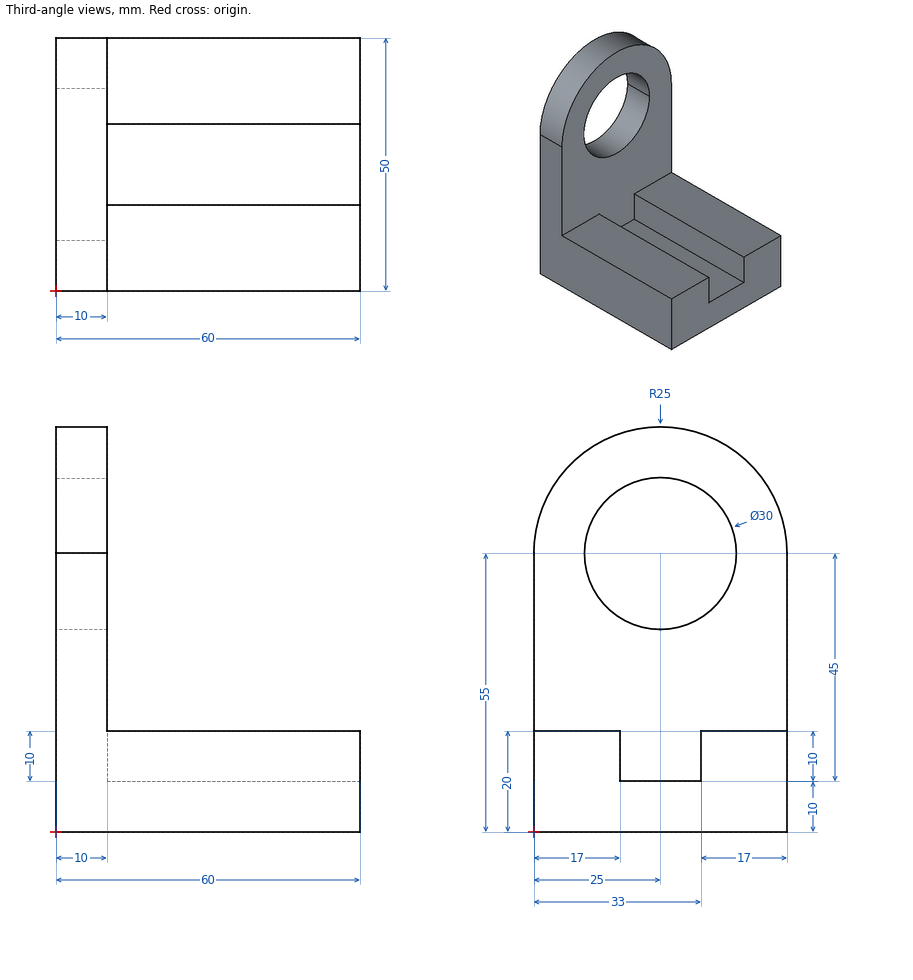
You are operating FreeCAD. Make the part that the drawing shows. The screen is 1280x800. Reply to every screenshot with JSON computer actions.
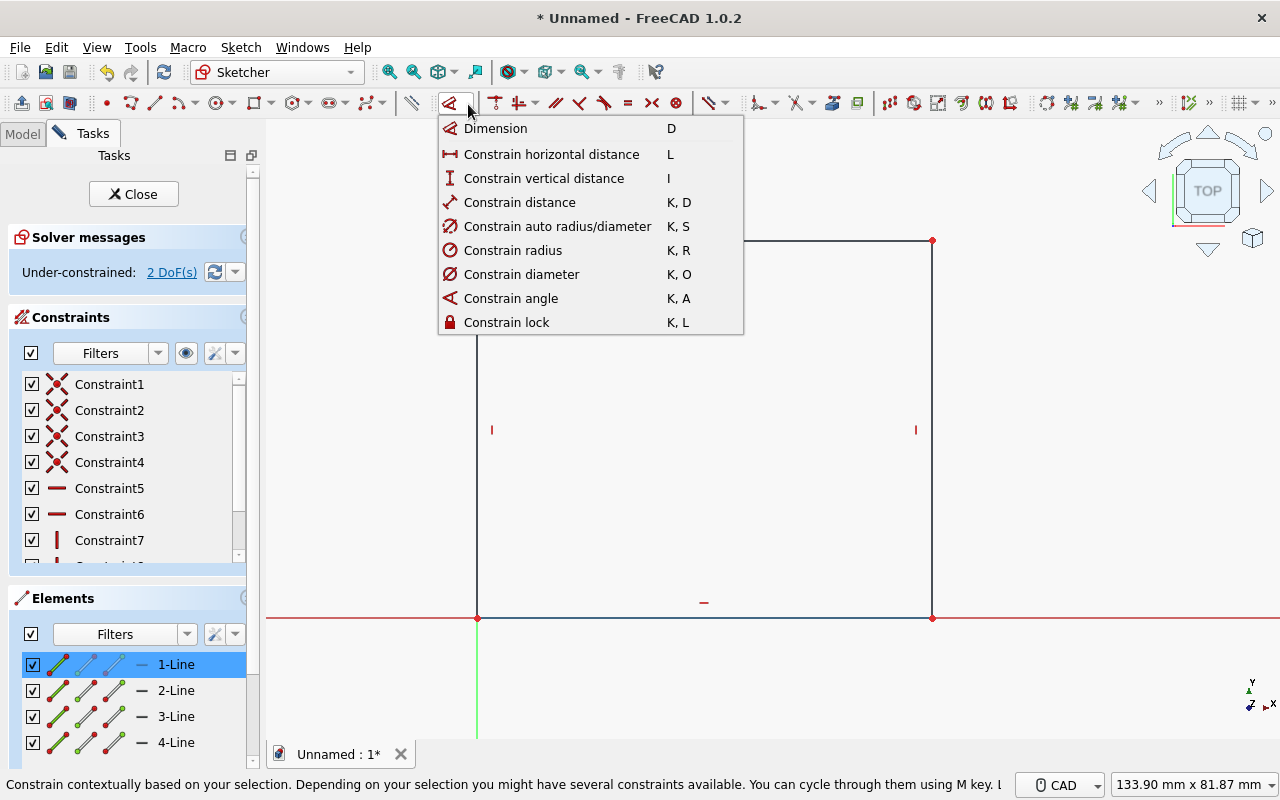
{"action": "left_click", "coordinate": [591, 154]}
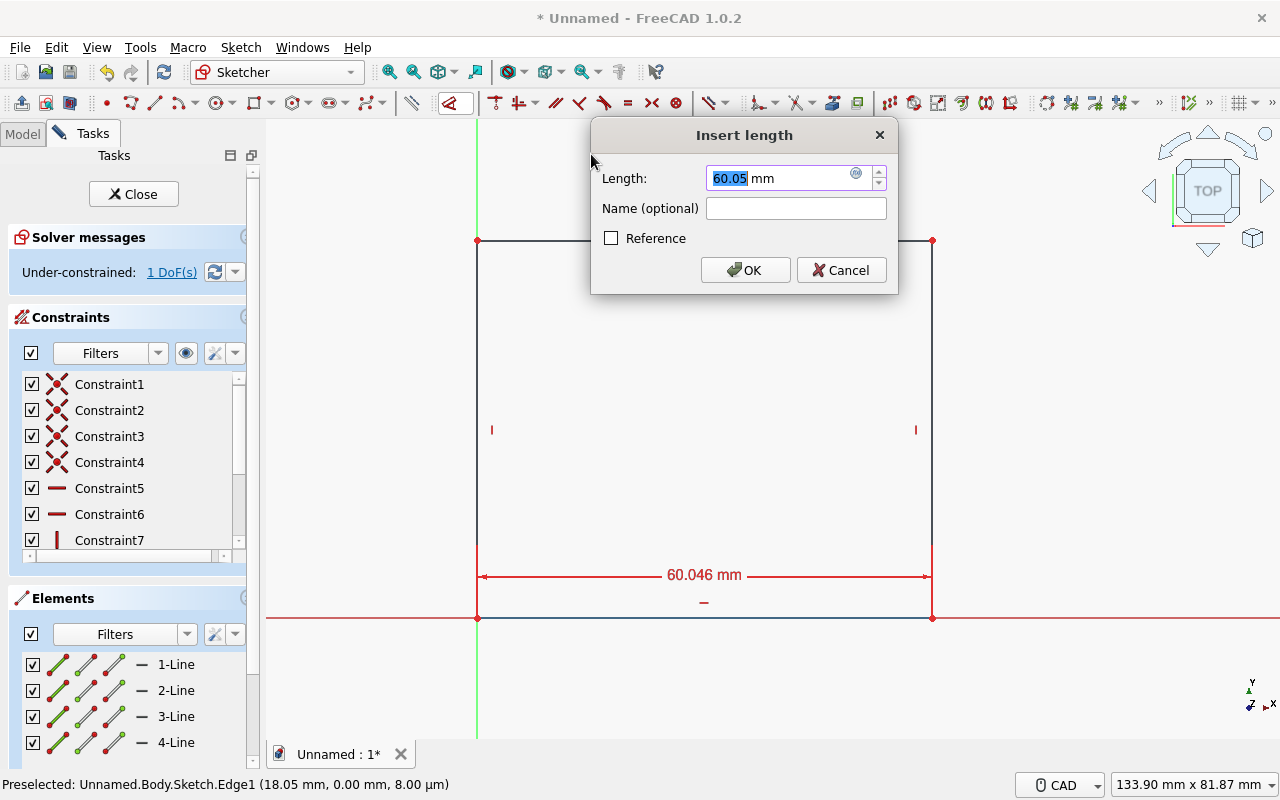
{"action": "type", "text": "60"}
{"action": "key", "text": "Return"}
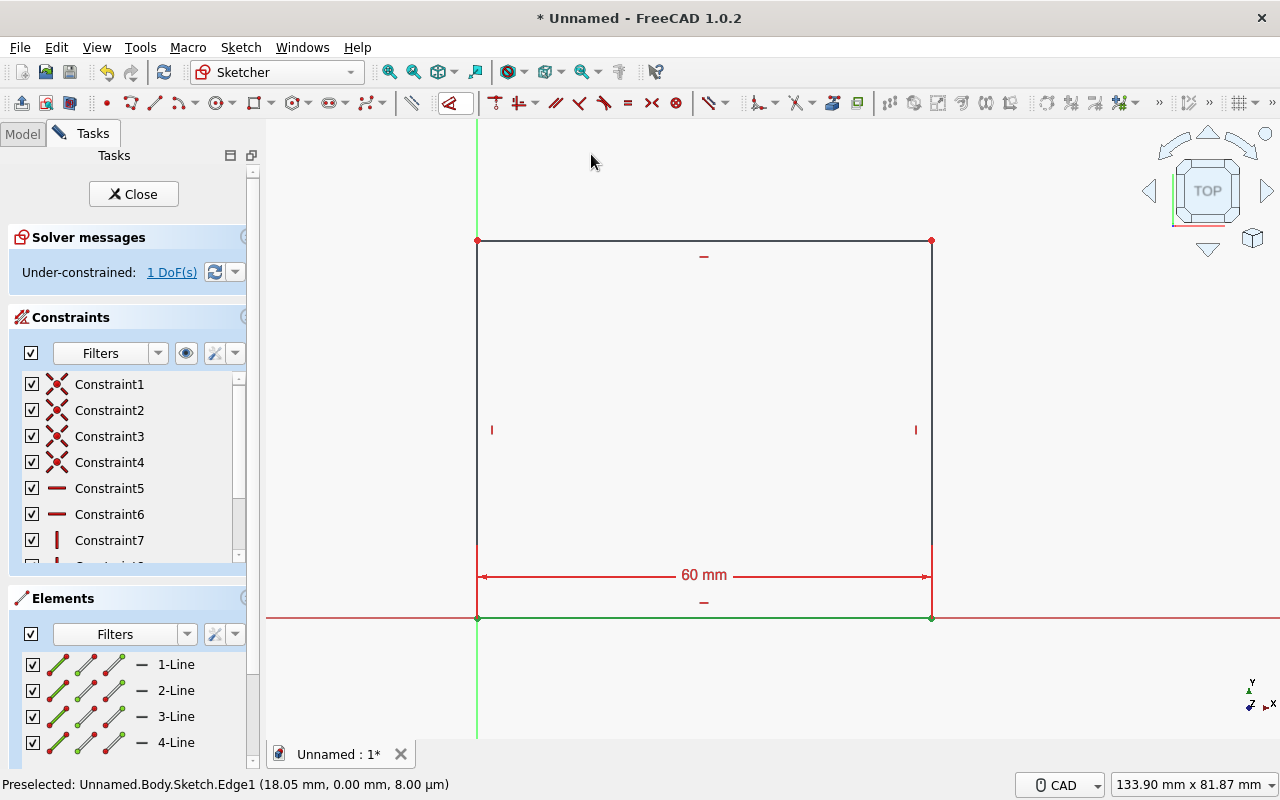
{"action": "left_click", "coordinate": [932, 505]}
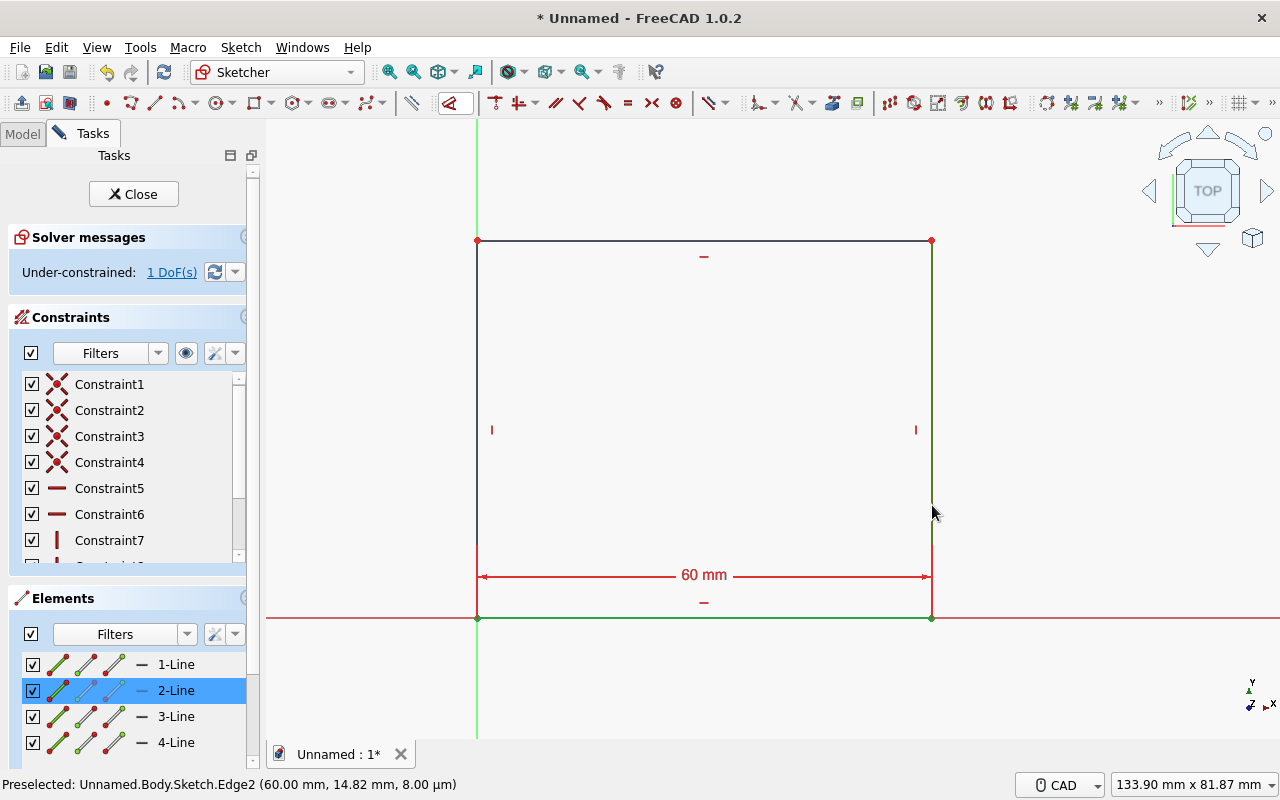
{"action": "left_click", "coordinate": [468, 104]}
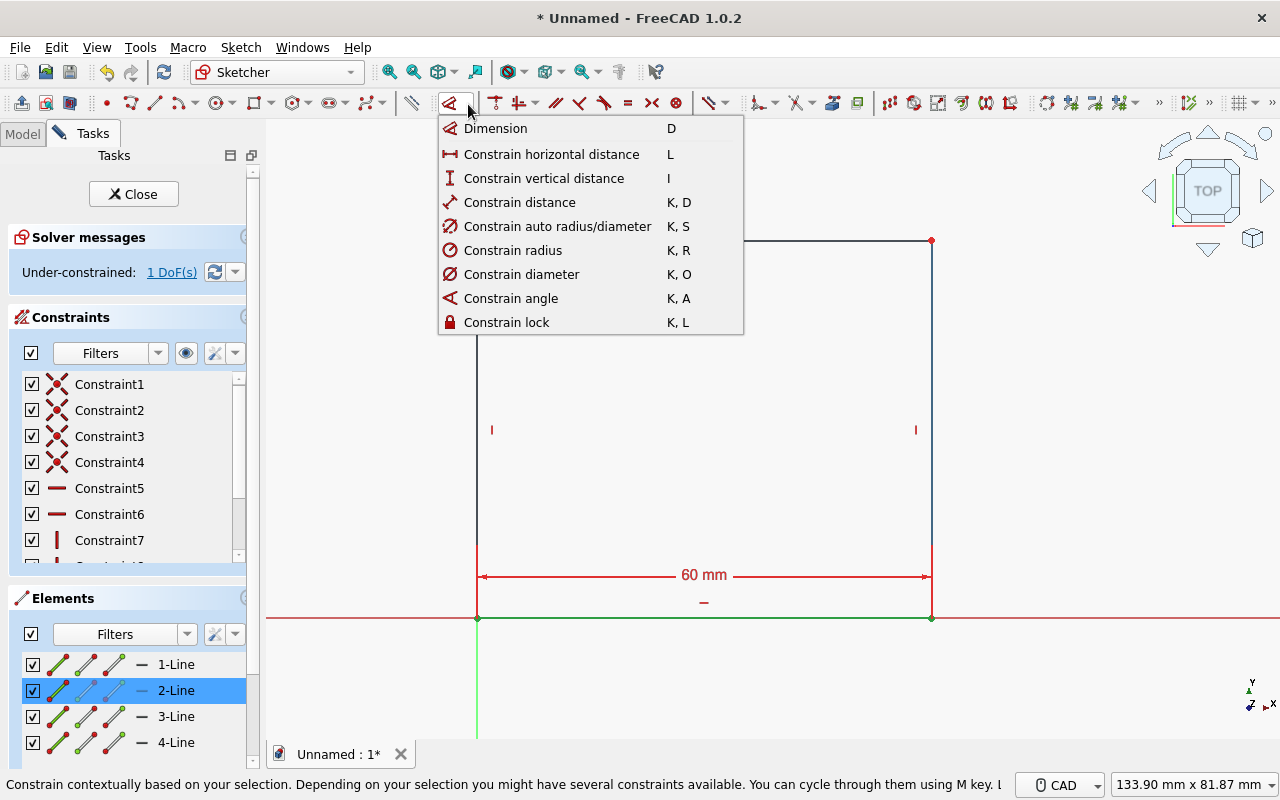
{"action": "left_click", "coordinate": [591, 178]}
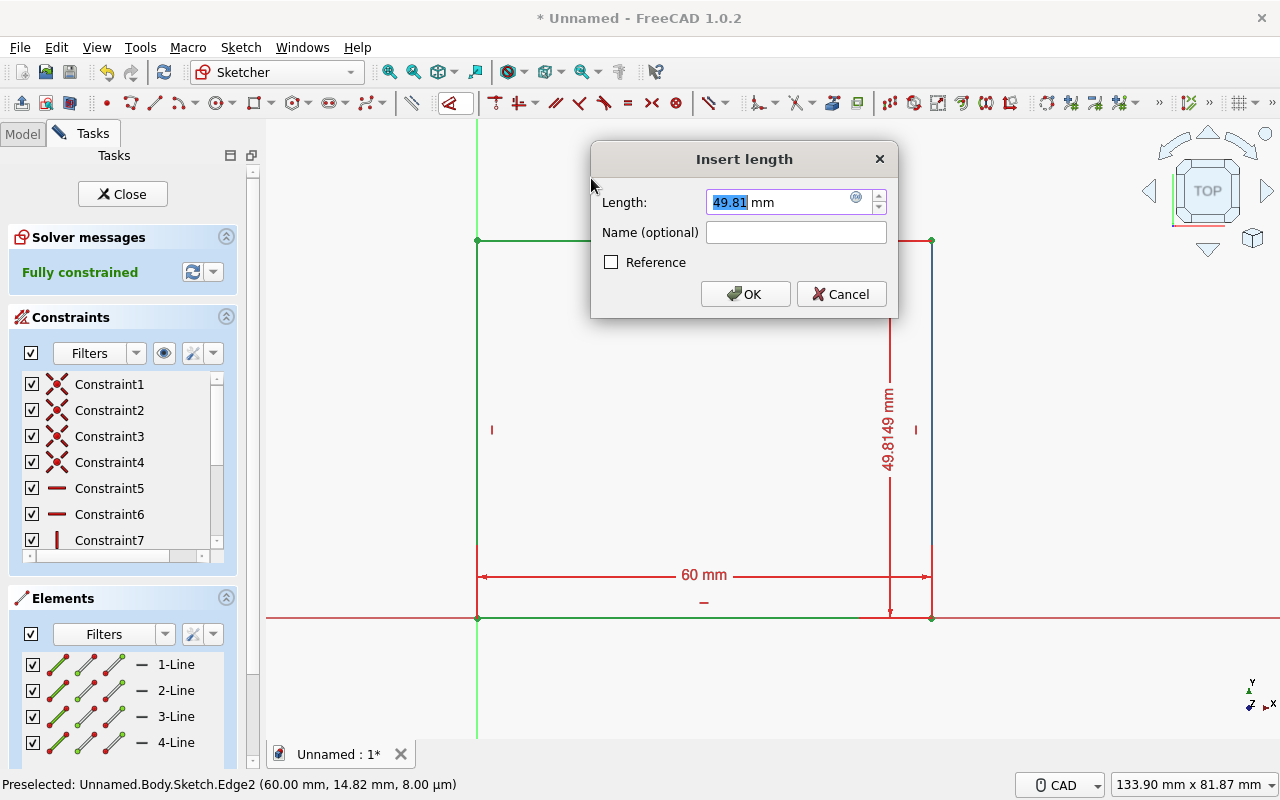
{"action": "type", "text": "50"}
{"action": "key", "text": "Return"}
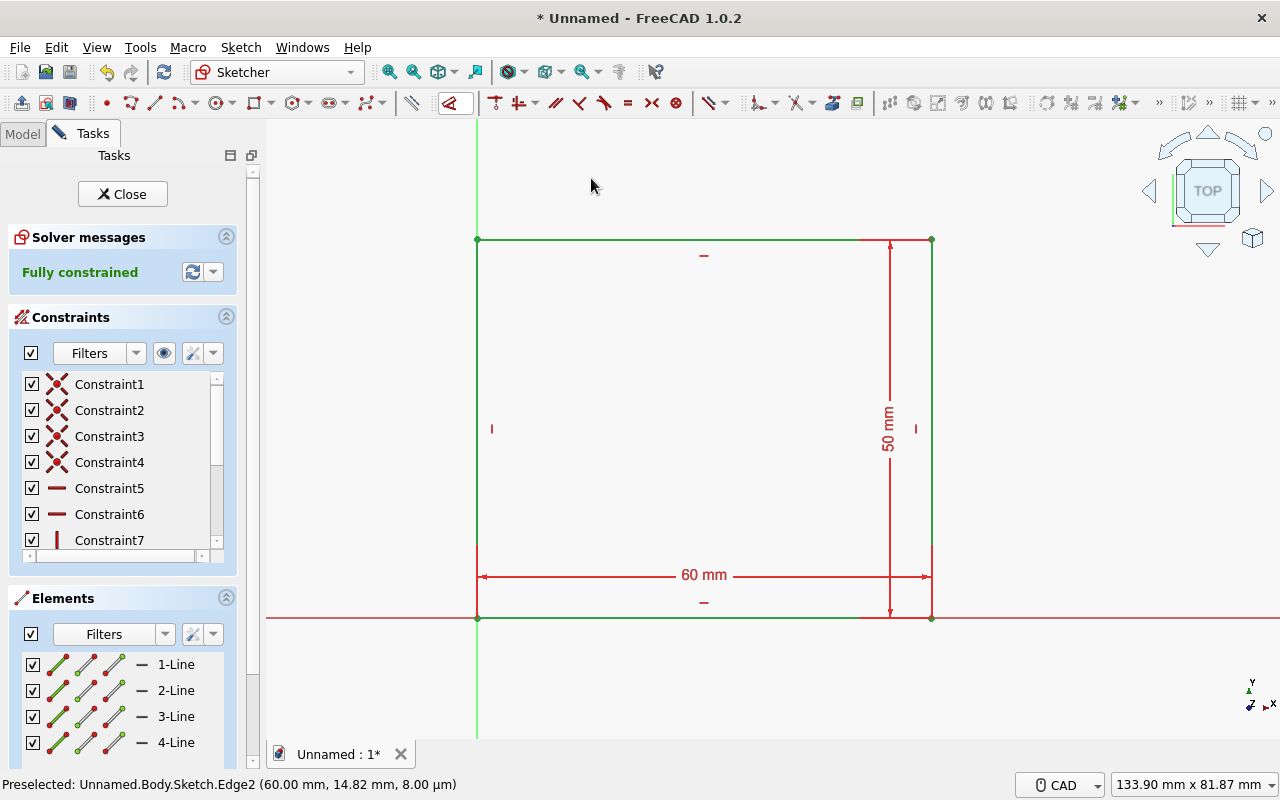
{"action": "left_click", "coordinate": [123, 194]}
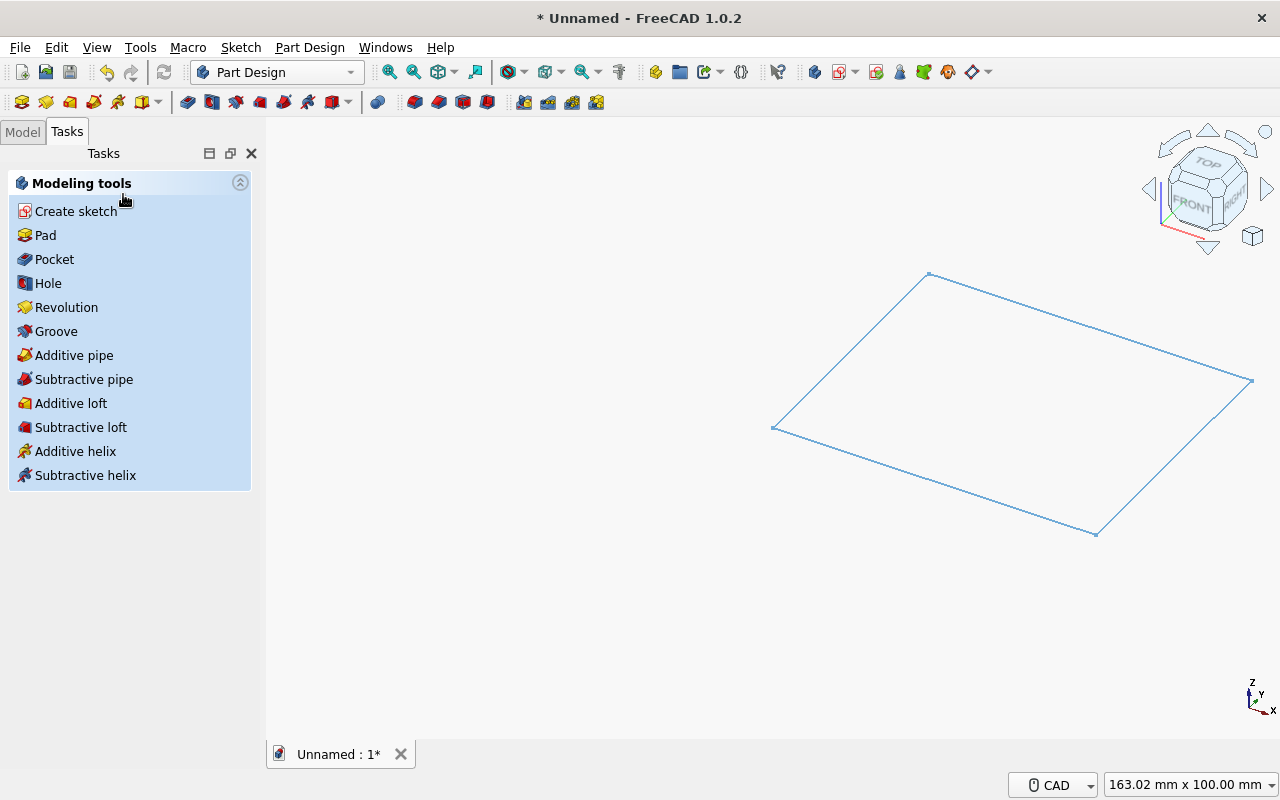
{"action": "left_click", "coordinate": [22, 102]}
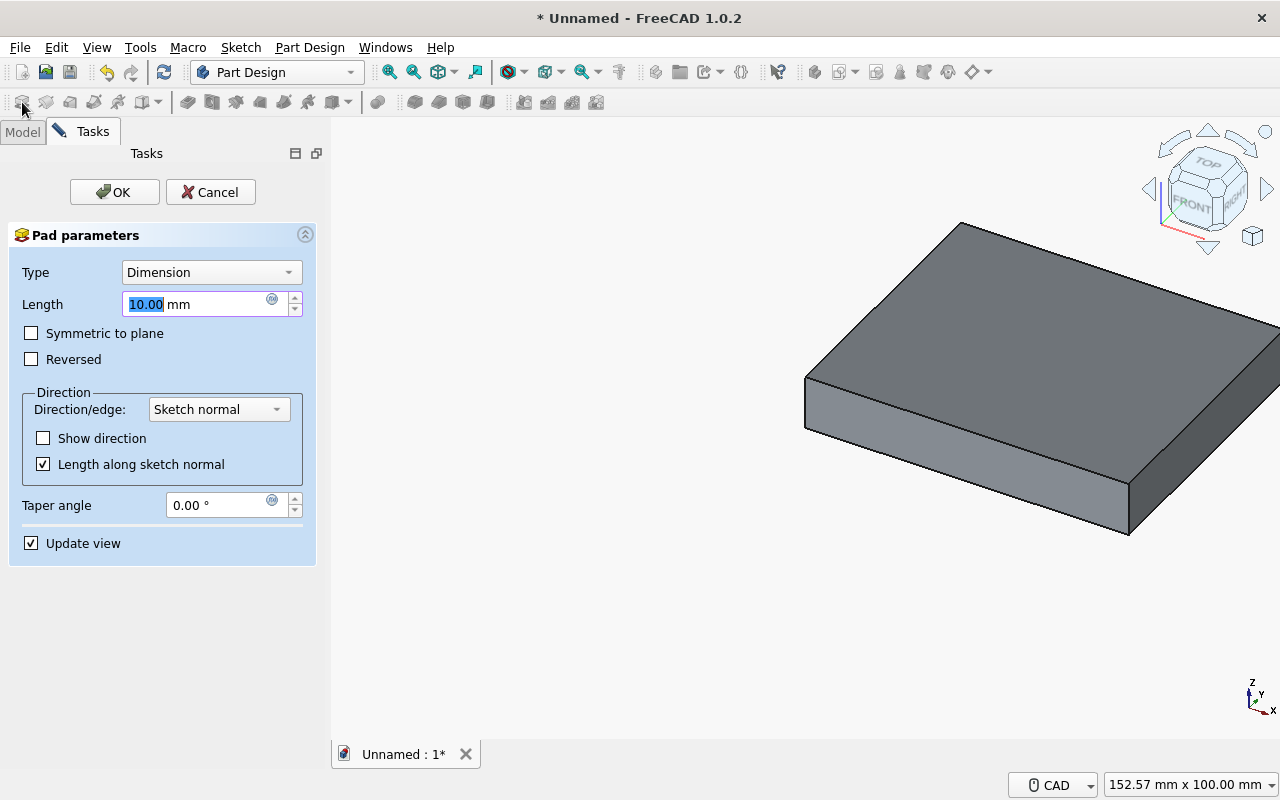
{"action": "type", "text": "10"}
{"action": "key", "text": "Tab"}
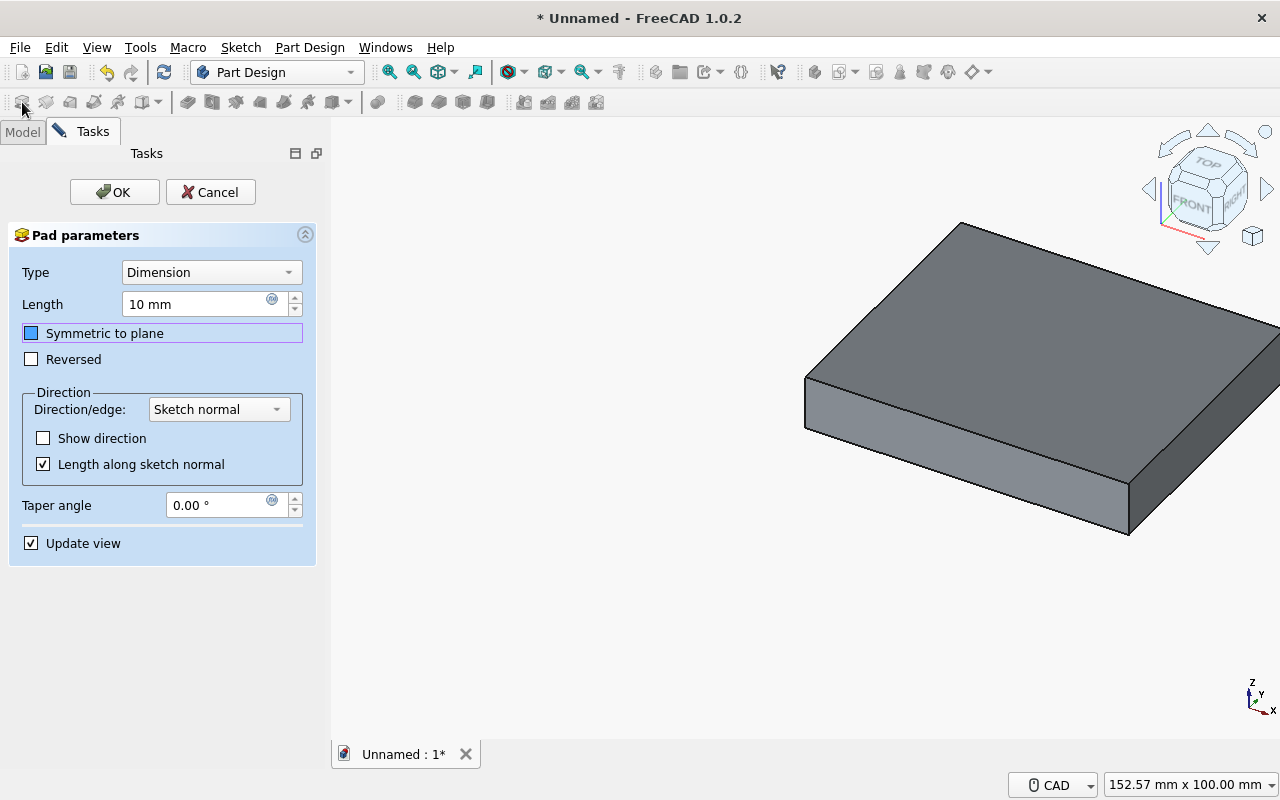
{"action": "left_click", "coordinate": [115, 192]}